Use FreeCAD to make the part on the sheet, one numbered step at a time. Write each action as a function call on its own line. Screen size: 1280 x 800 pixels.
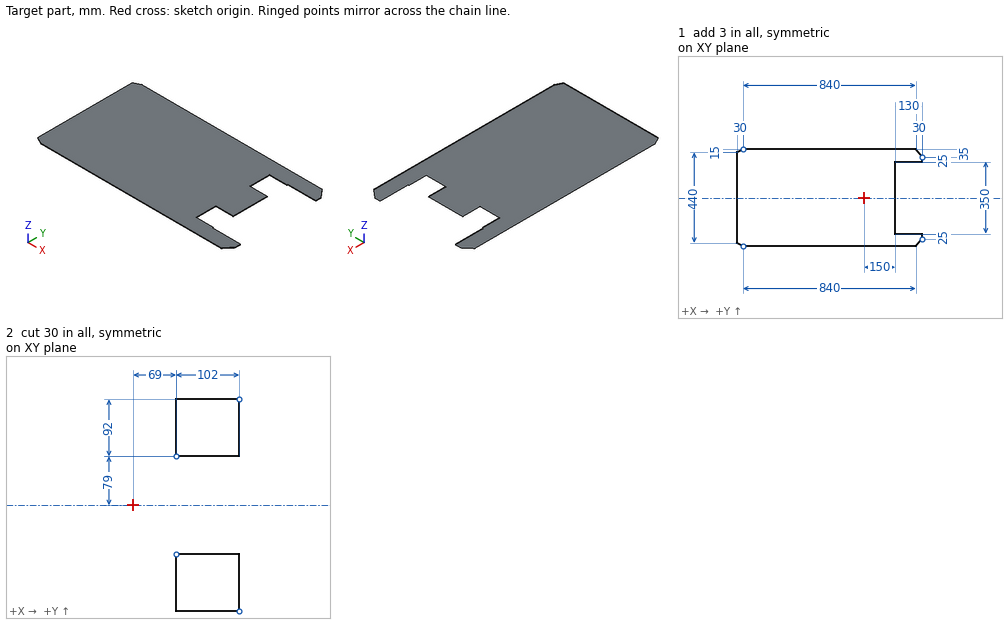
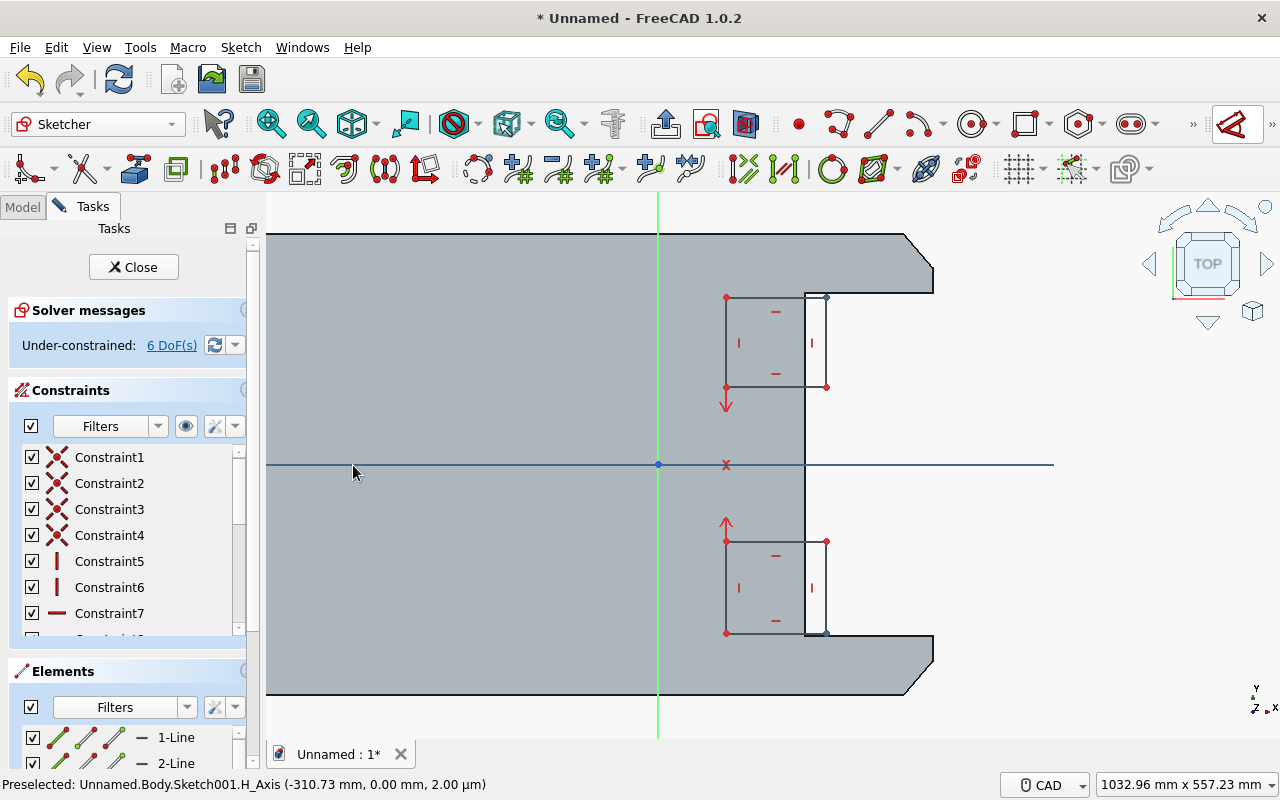
key(s)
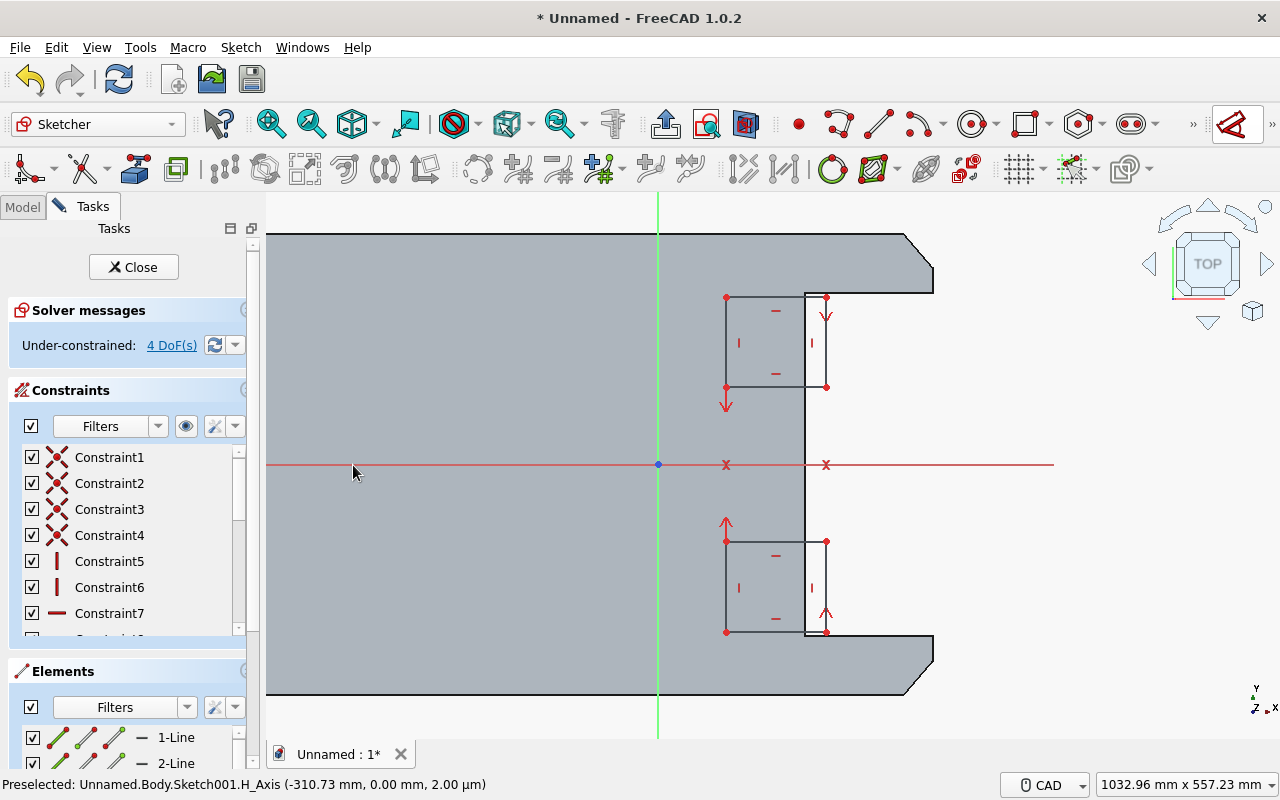
click(1232, 124)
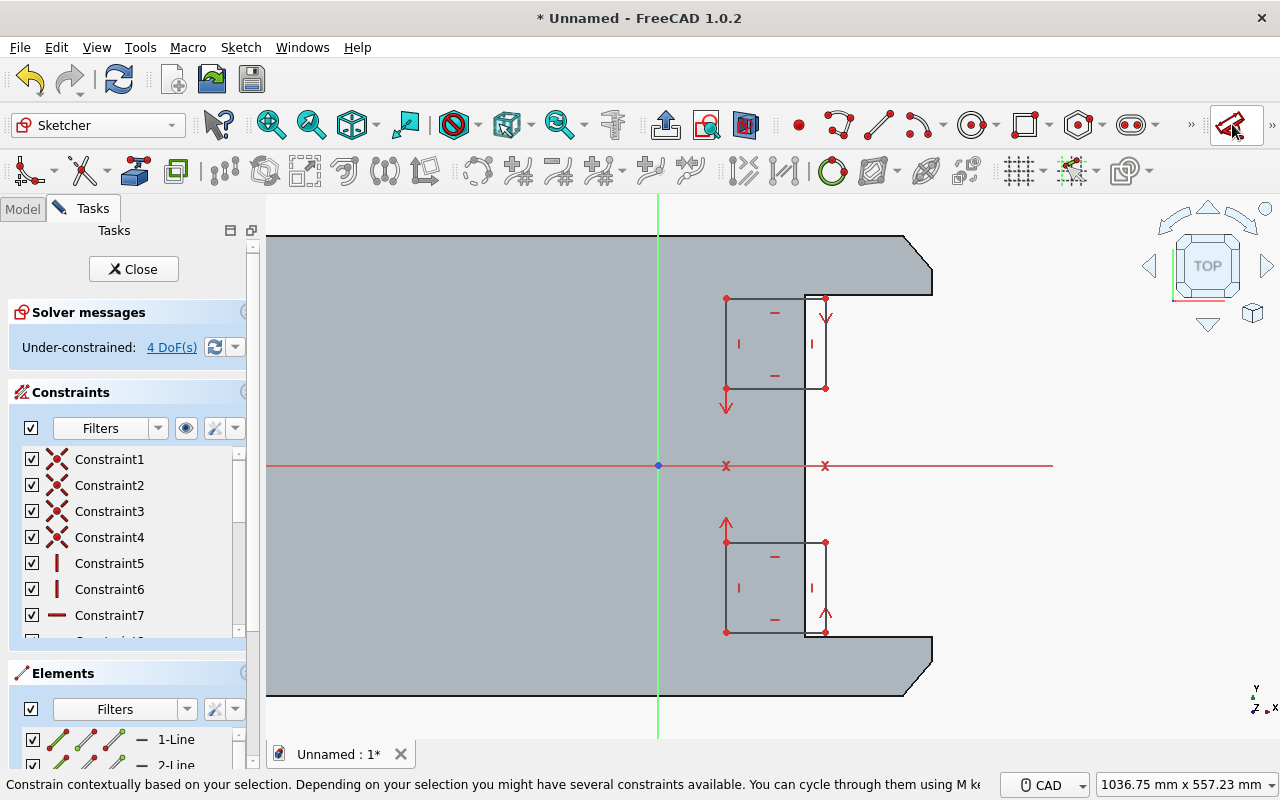
click(726, 326)
click(692, 344)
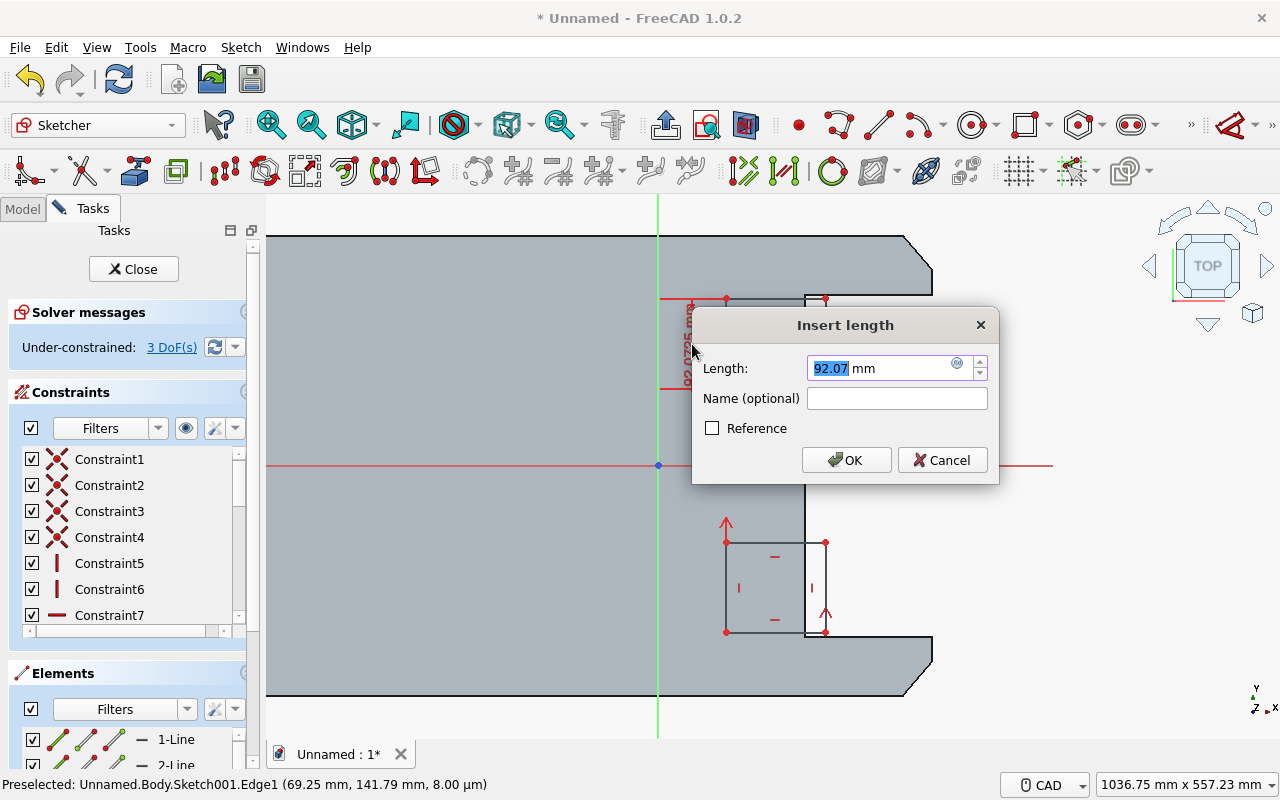
text(92)
key(Return)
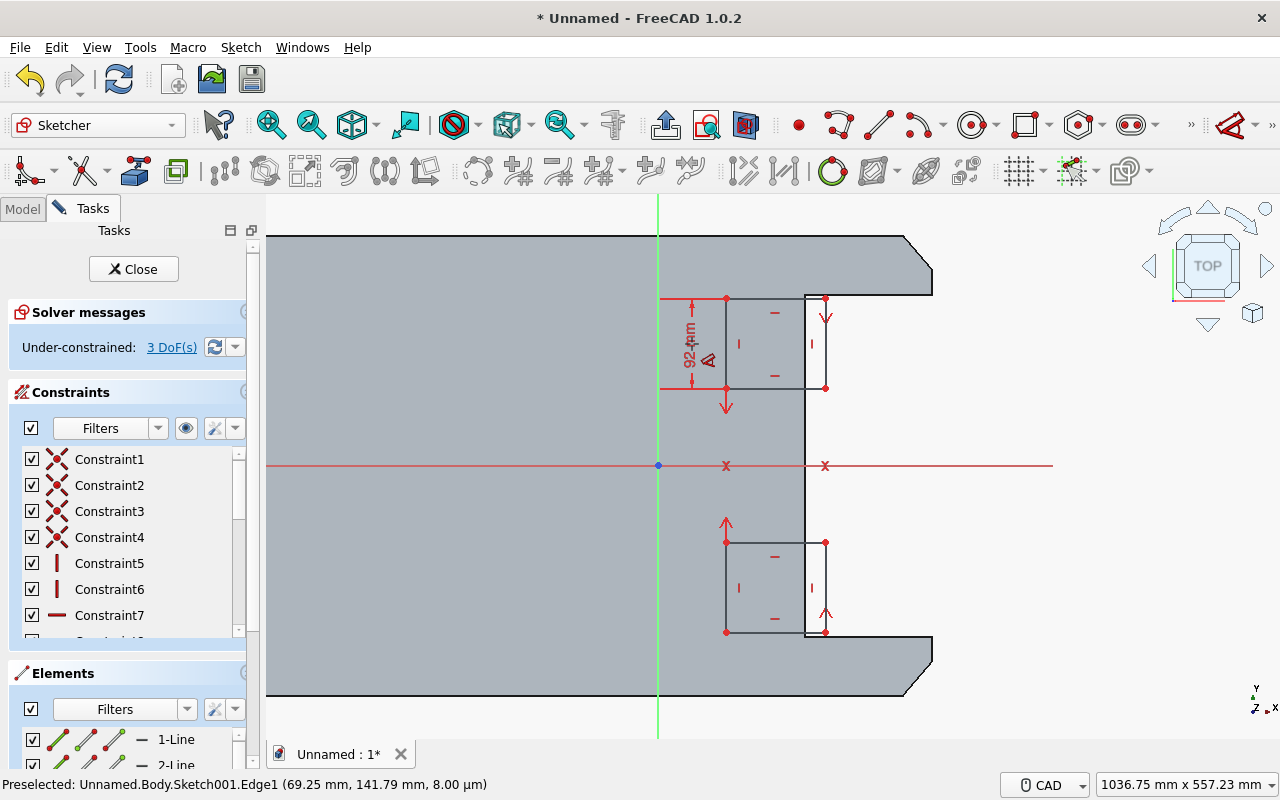
click(756, 389)
click(776, 355)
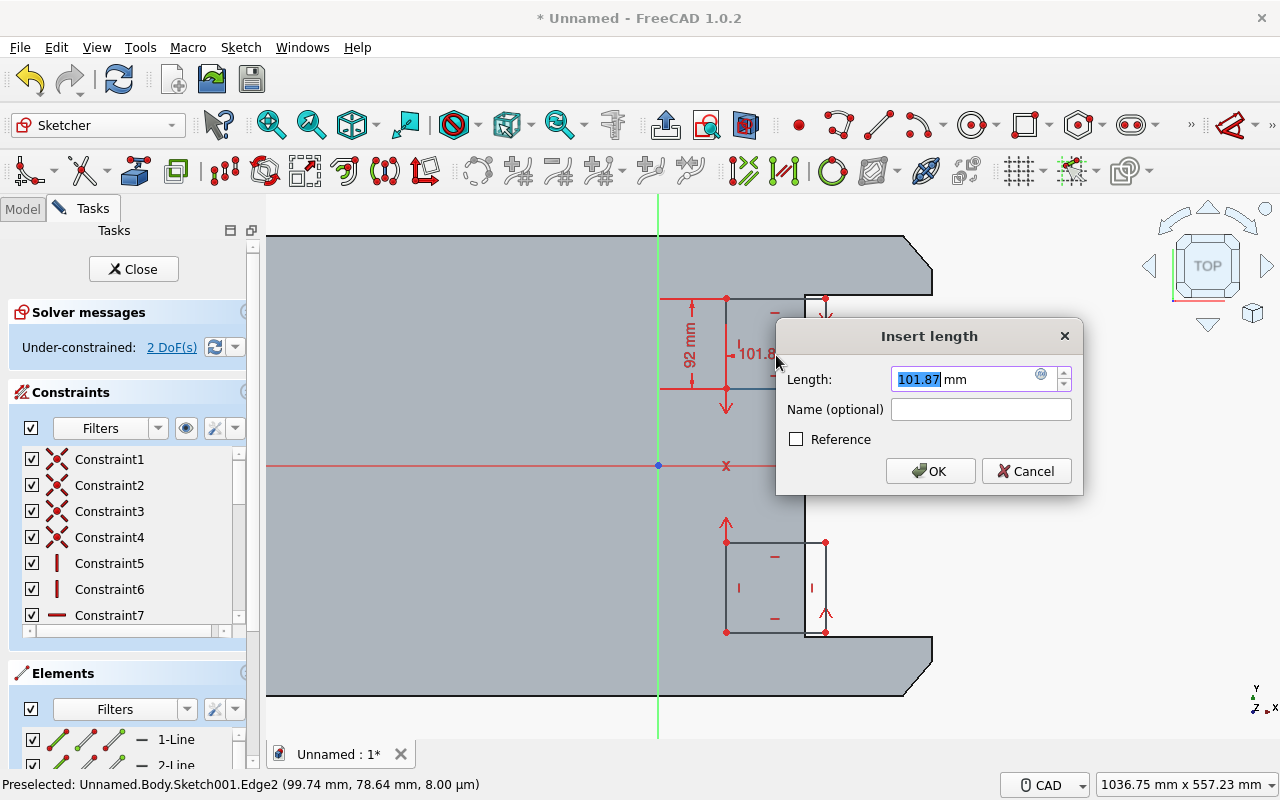
text(102)
key(Return)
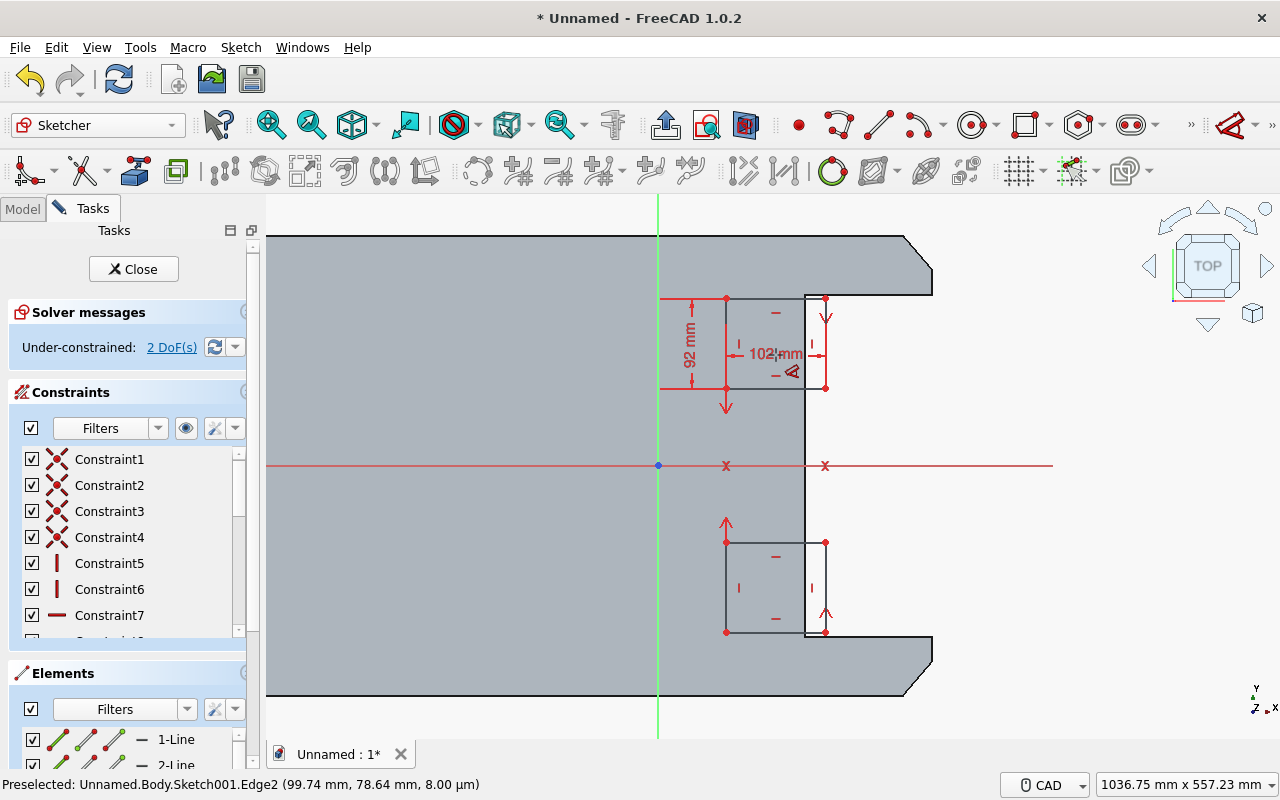
click(726, 299)
click(692, 265)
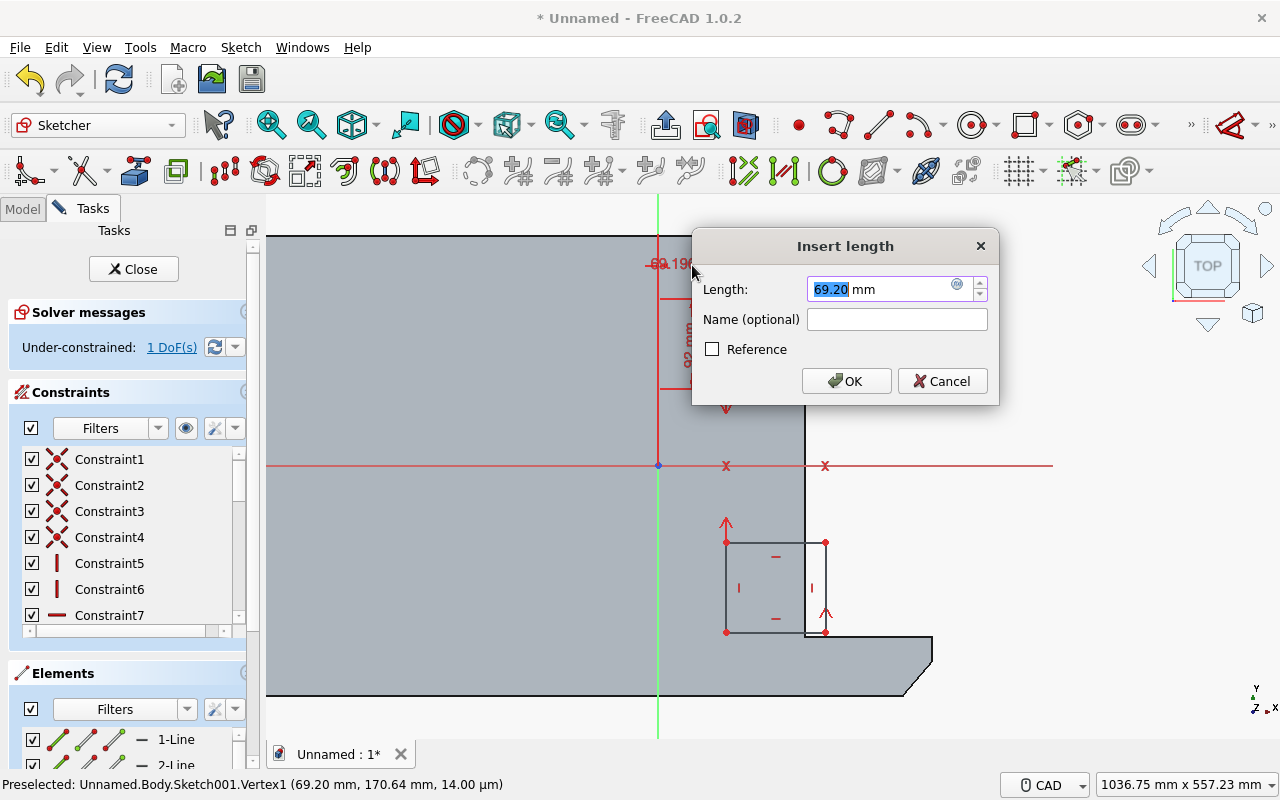
text(69)
key(Return)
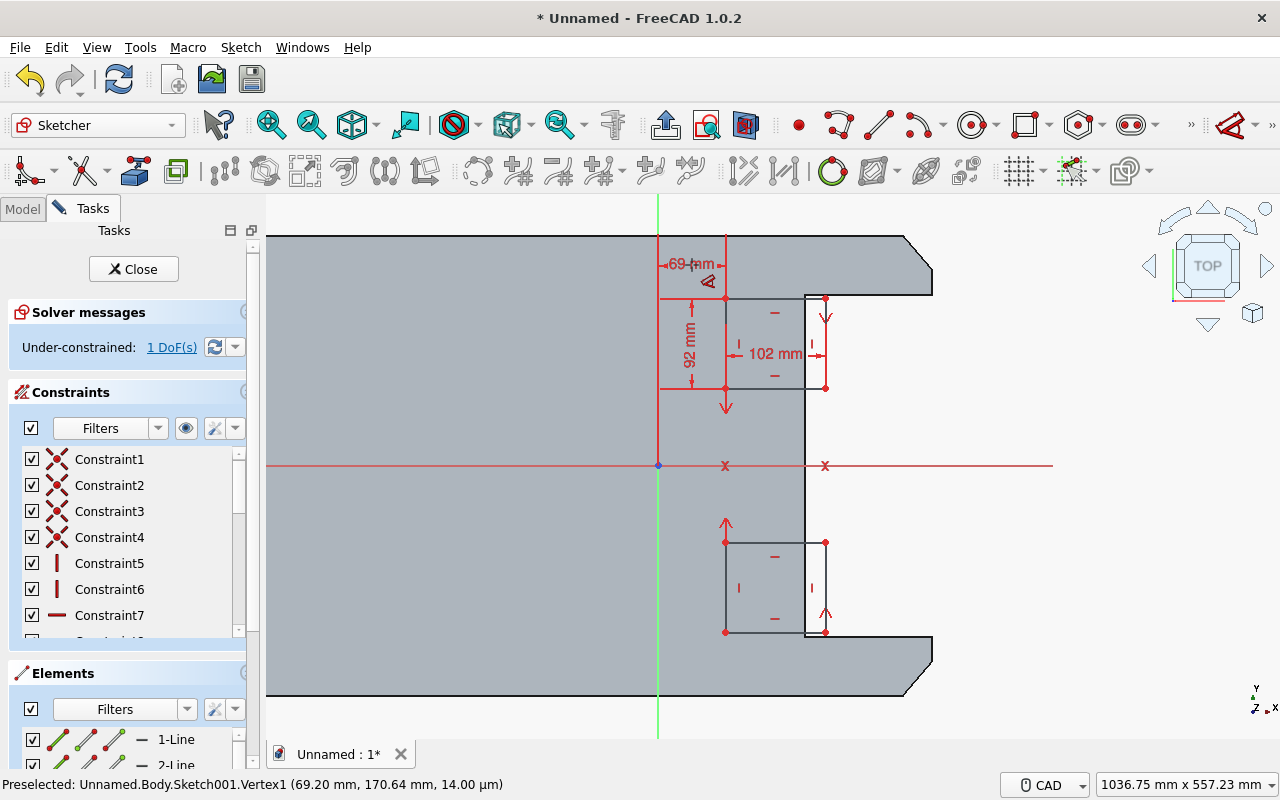
click(726, 389)
click(624, 427)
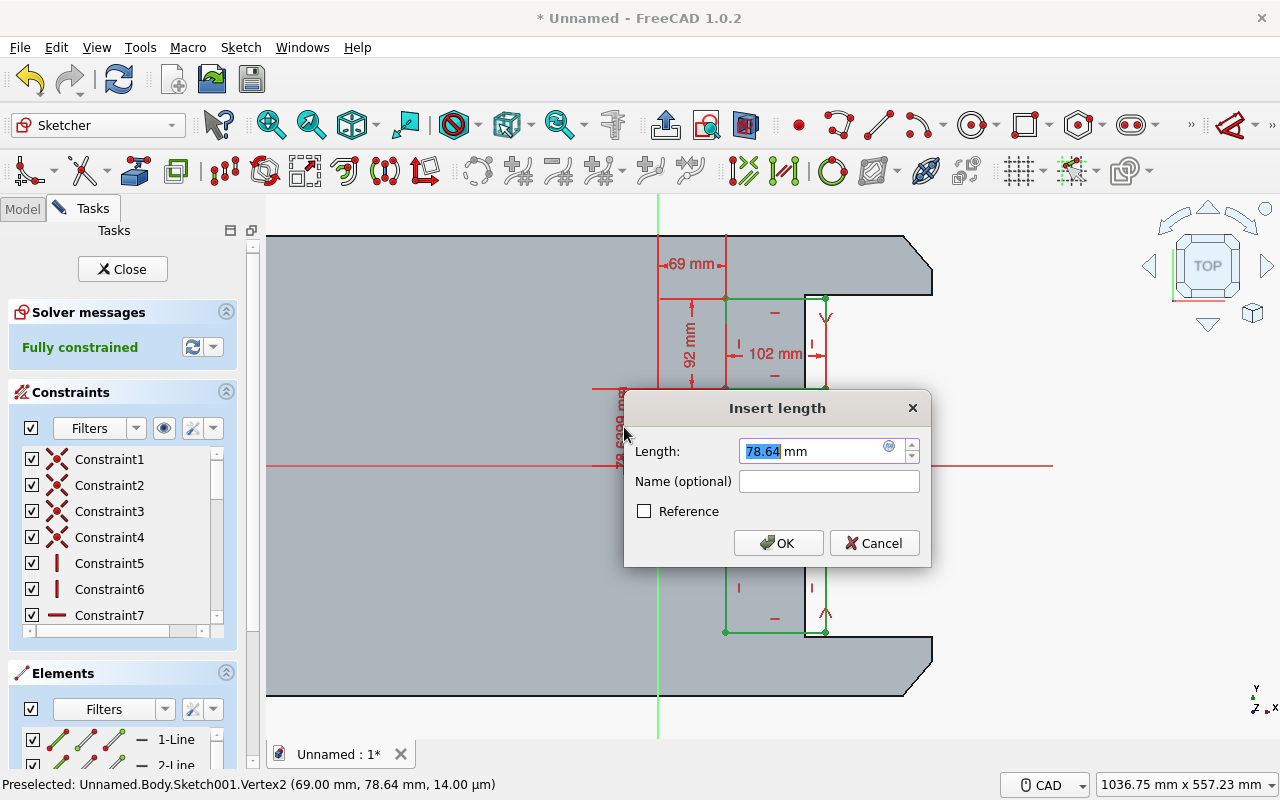
text(79)
key(Return)
key(Escape)